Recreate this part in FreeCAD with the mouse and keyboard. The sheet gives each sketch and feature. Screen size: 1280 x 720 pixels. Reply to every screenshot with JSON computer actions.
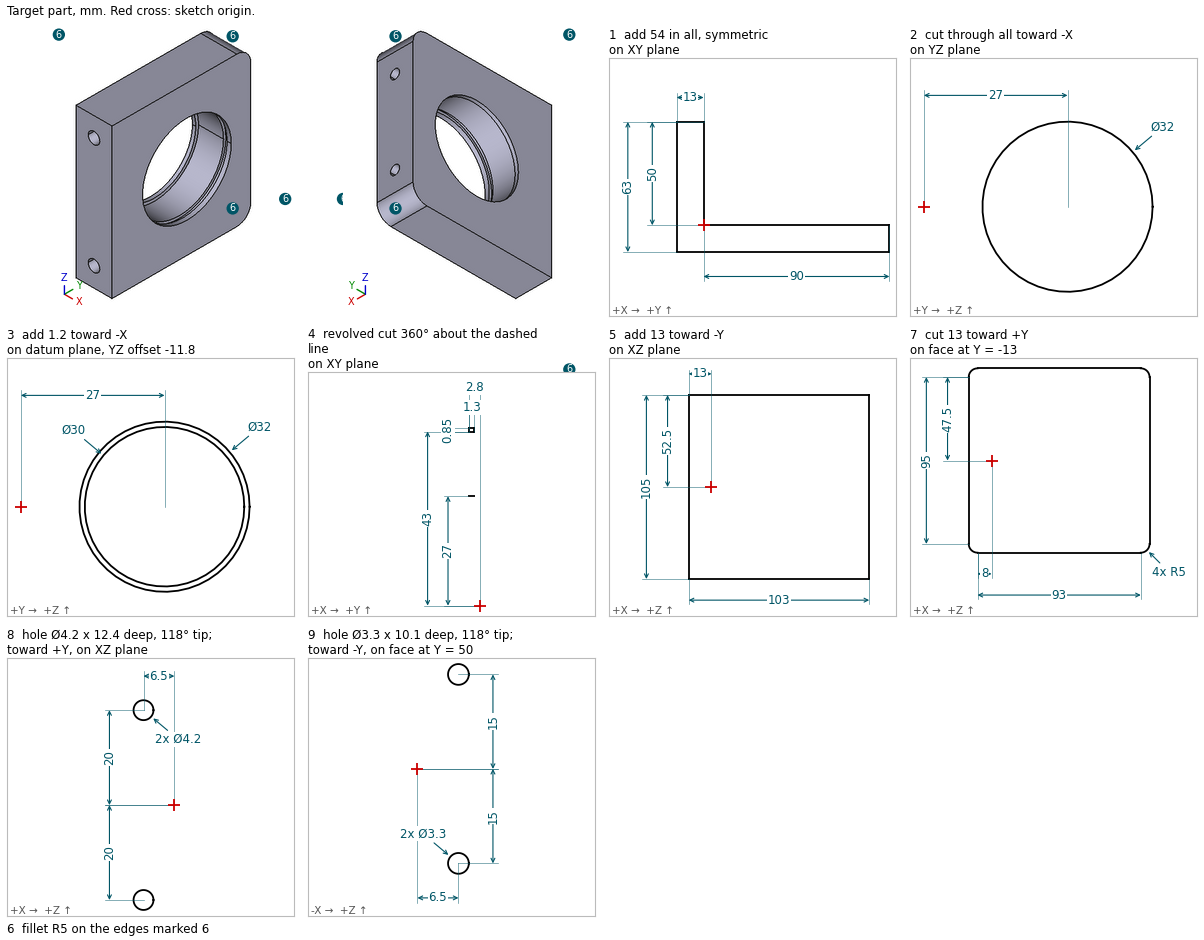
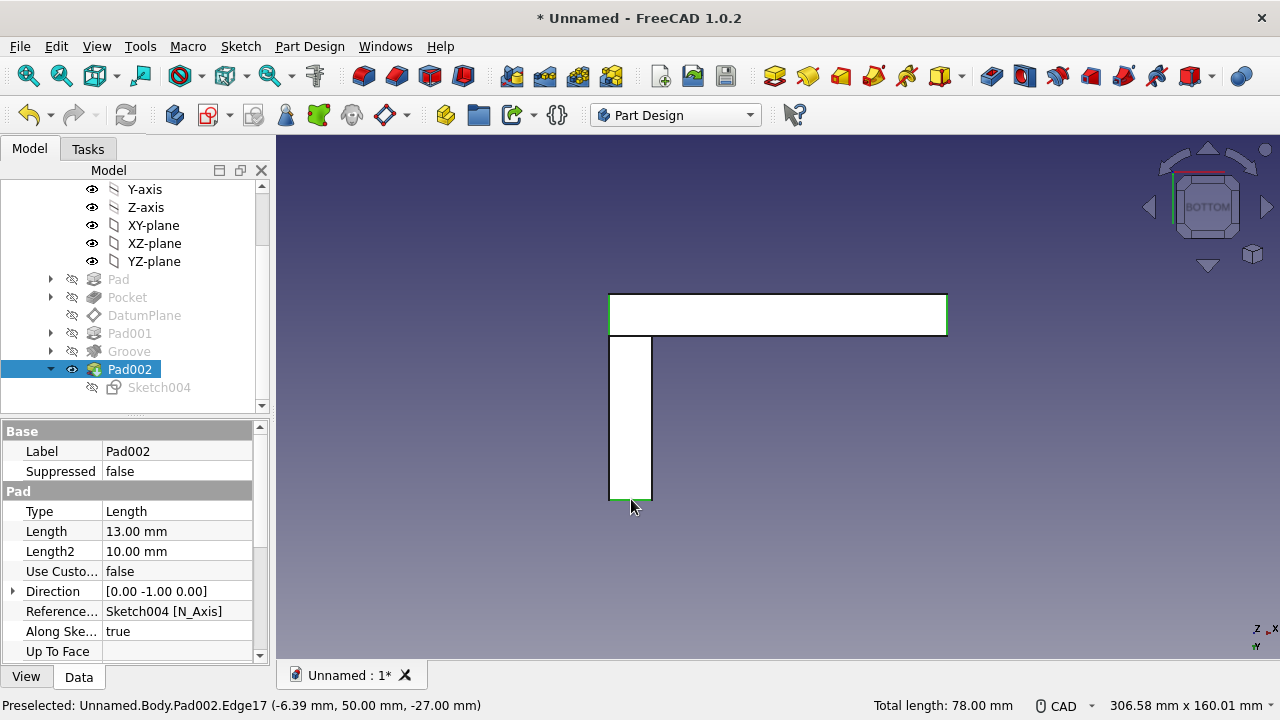
{"action": "left_click", "coordinate": [364, 76]}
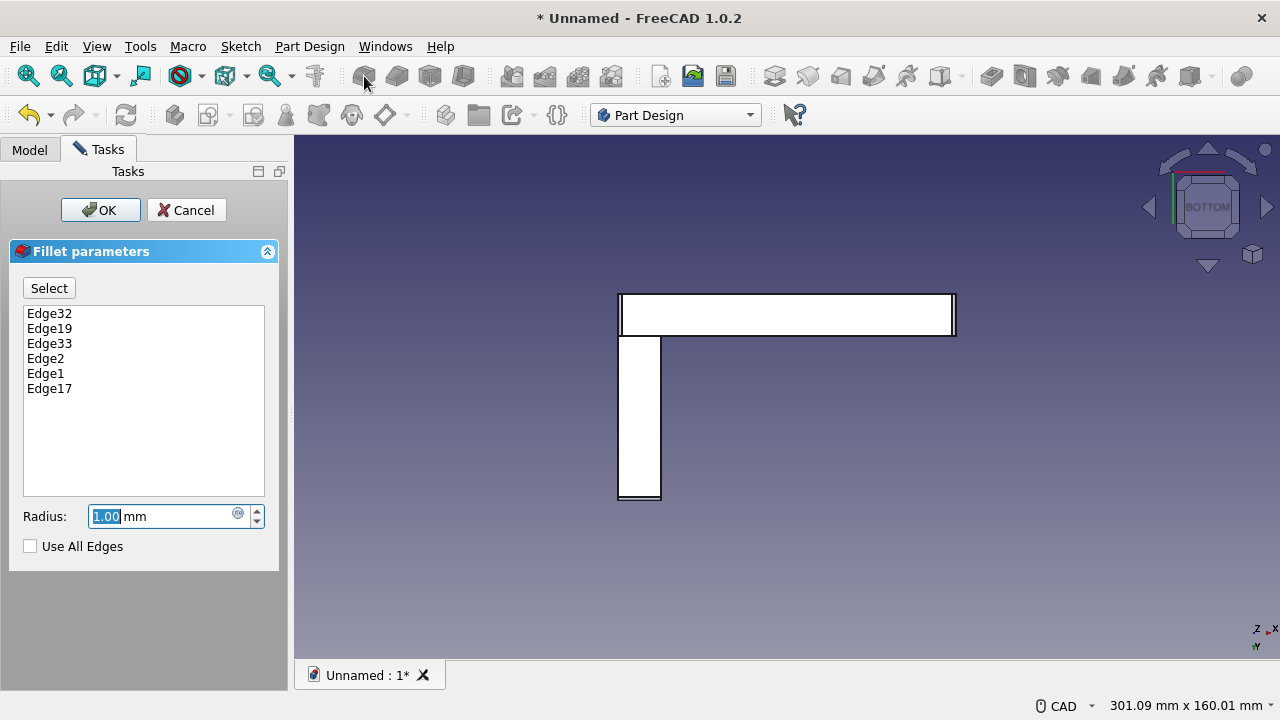
{"action": "type", "text": "5"}
{"action": "key", "text": "Tab"}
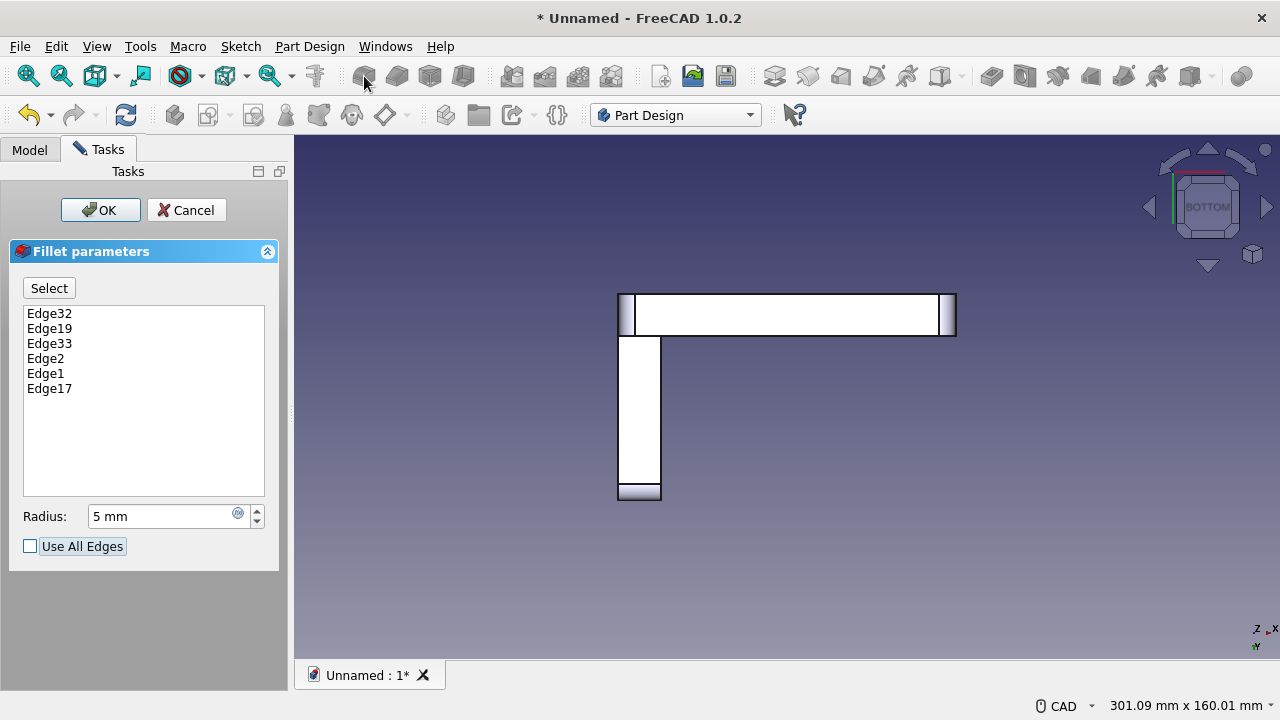
{"action": "left_click", "coordinate": [101, 210]}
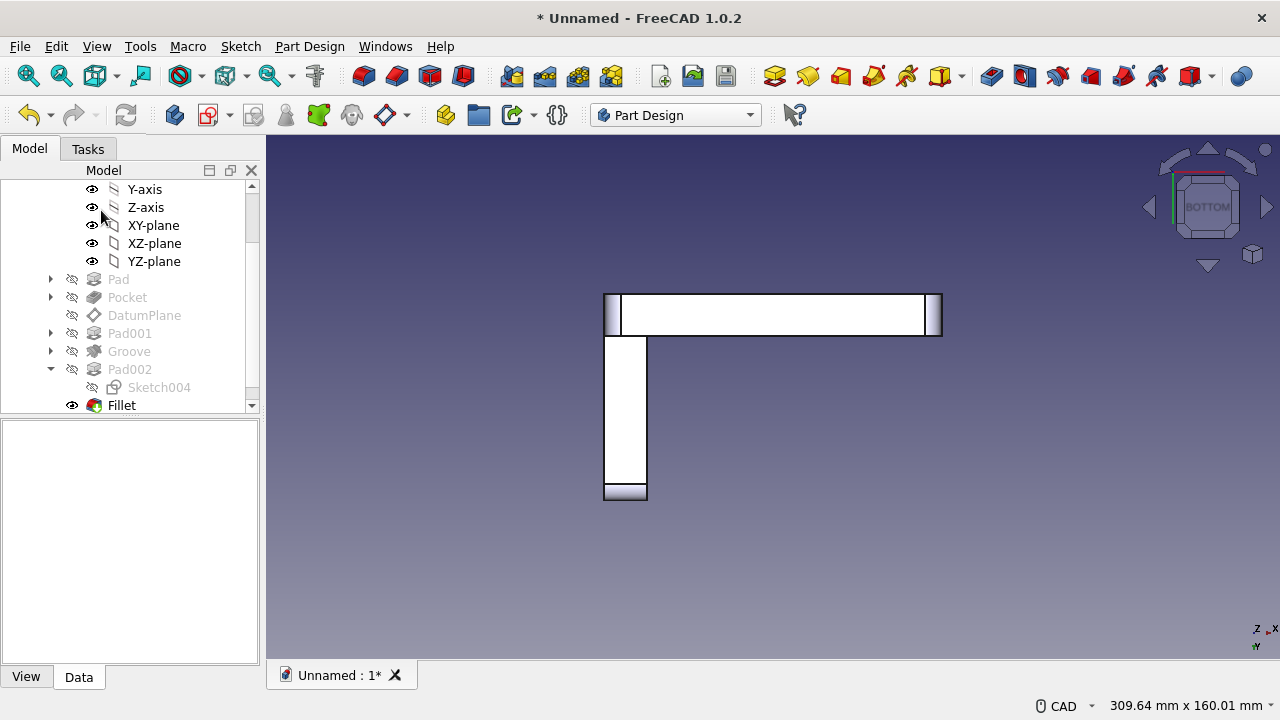
{"action": "left_click", "coordinate": [29, 76]}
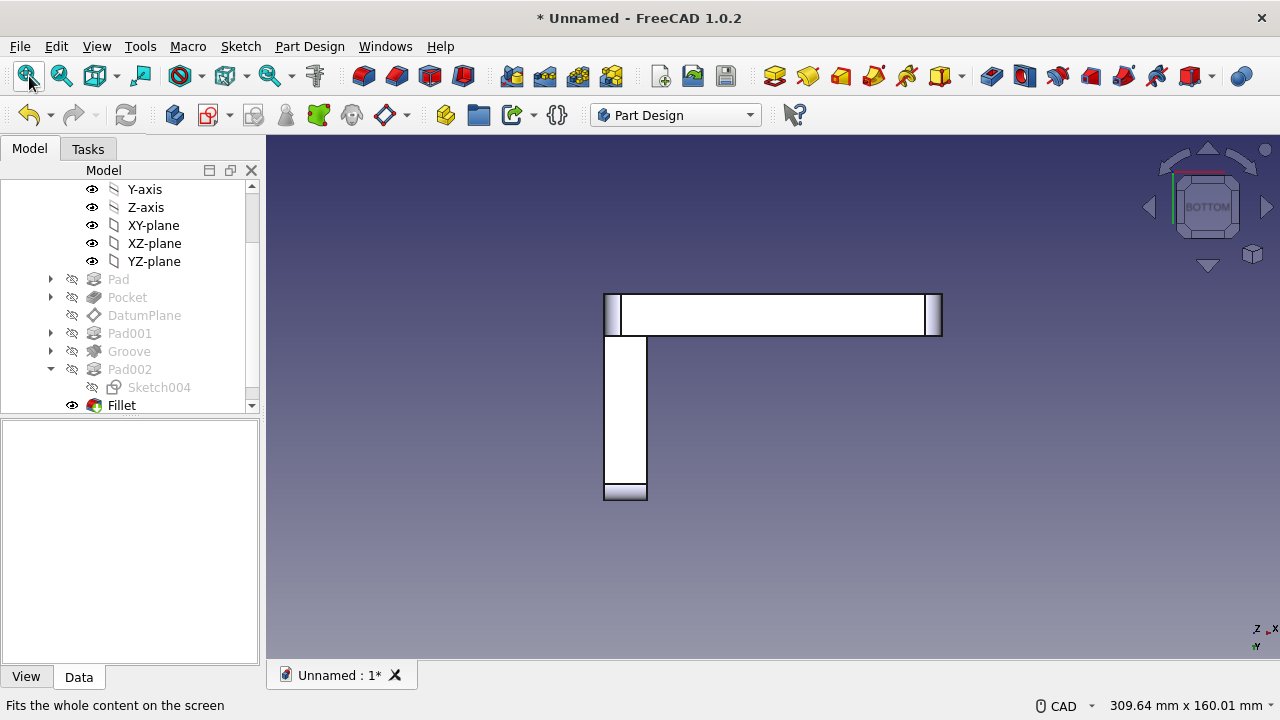
{"action": "key", "text": "0"}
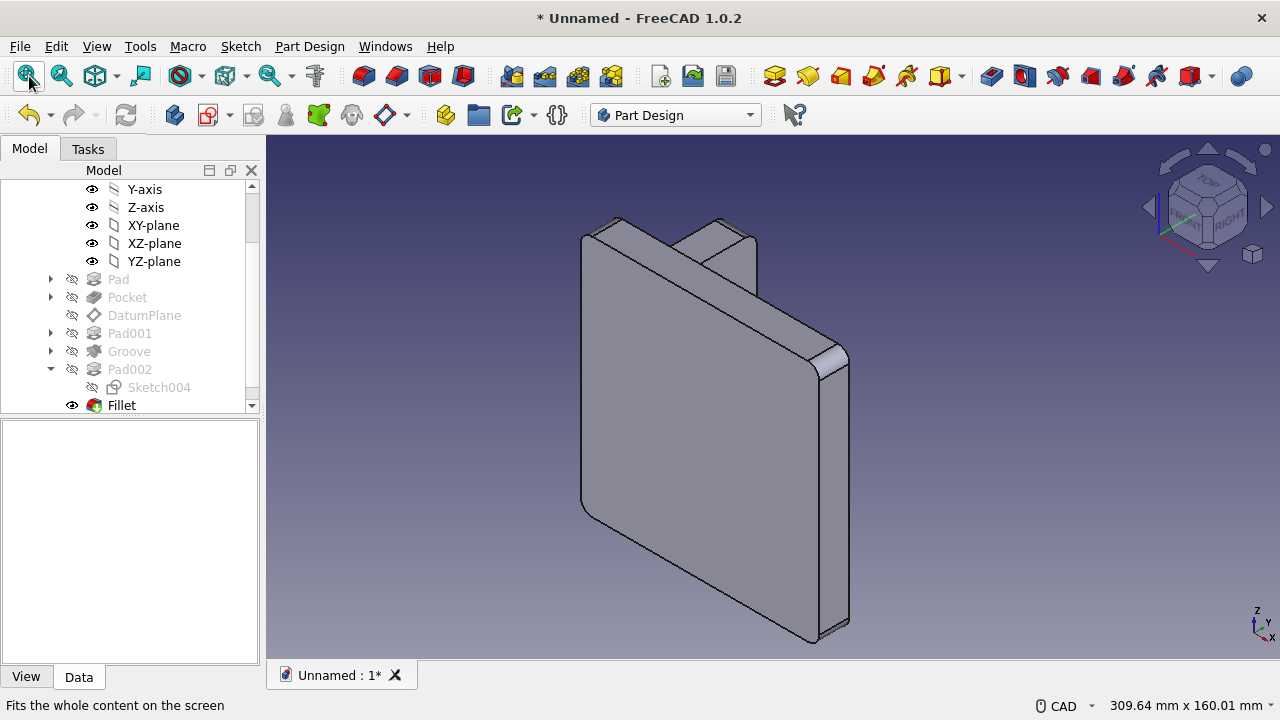
{"action": "left_click", "coordinate": [700, 438]}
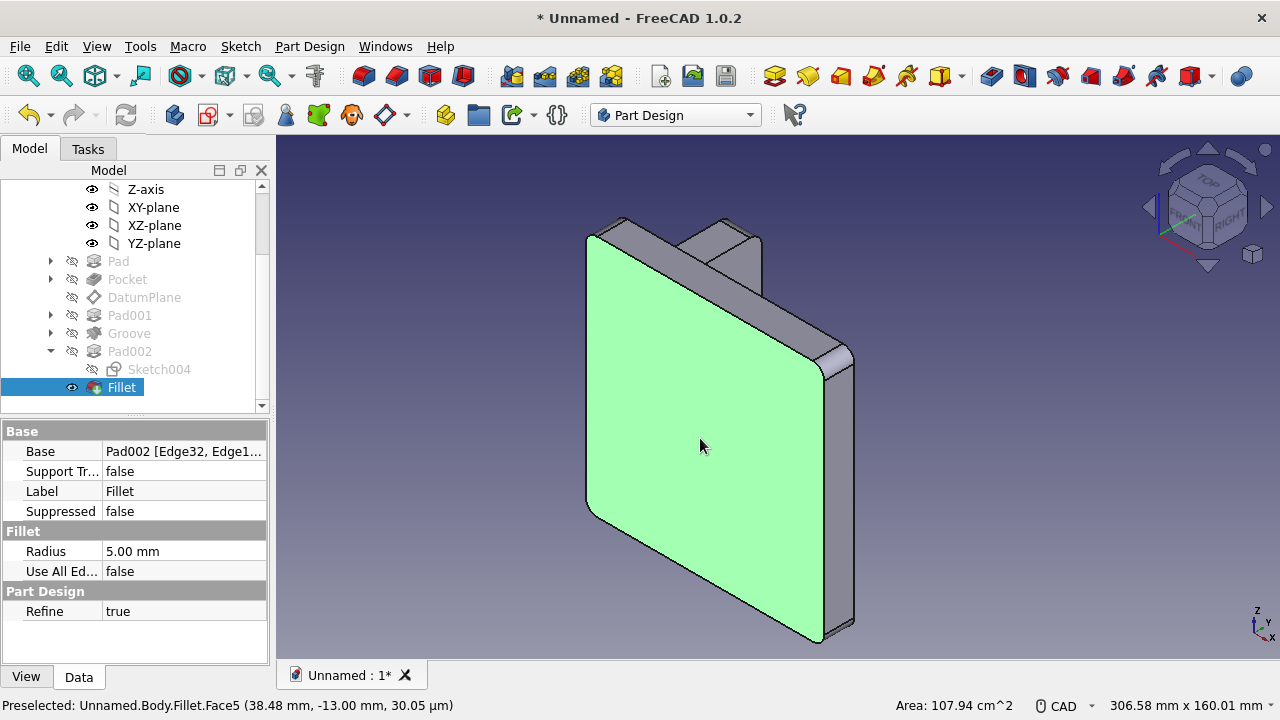
{"action": "left_click", "coordinate": [208, 116]}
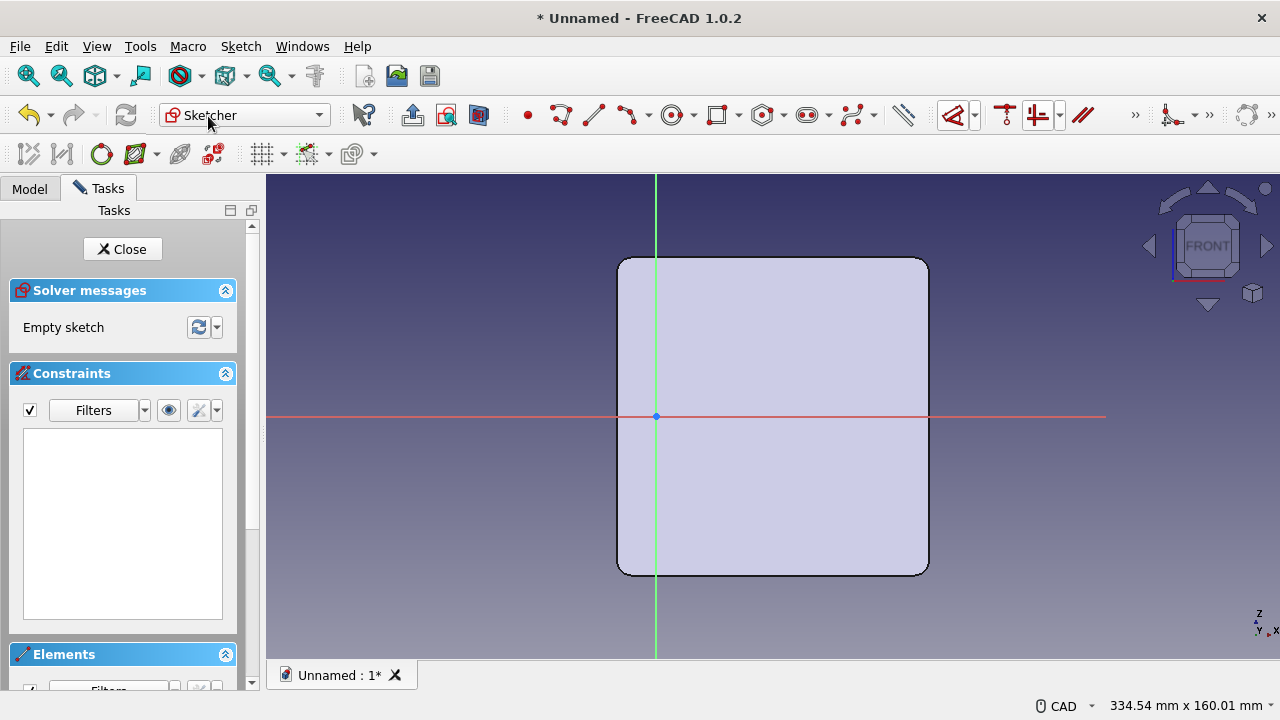
{"action": "left_click", "coordinate": [594, 116]}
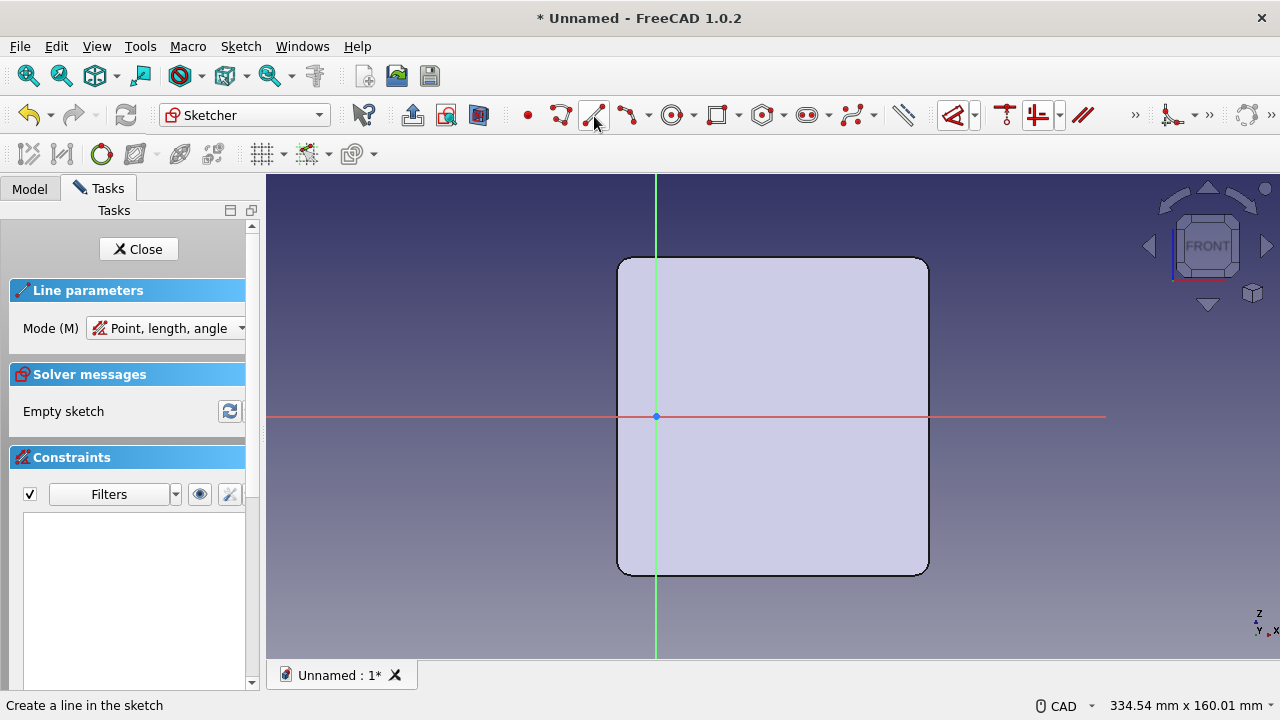
{"action": "left_click", "coordinate": [617, 273]}
{"action": "left_click", "coordinate": [617, 560]}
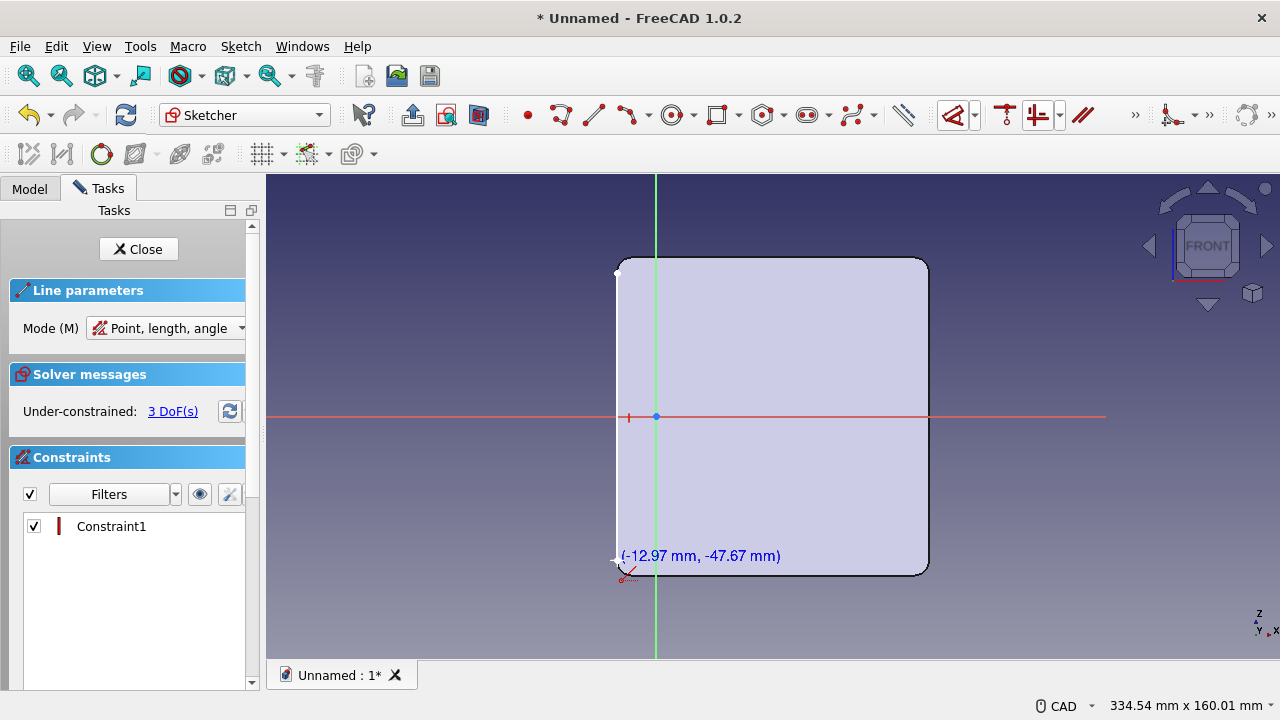
{"action": "left_click", "coordinate": [632, 576]}
{"action": "left_click", "coordinate": [914, 576]}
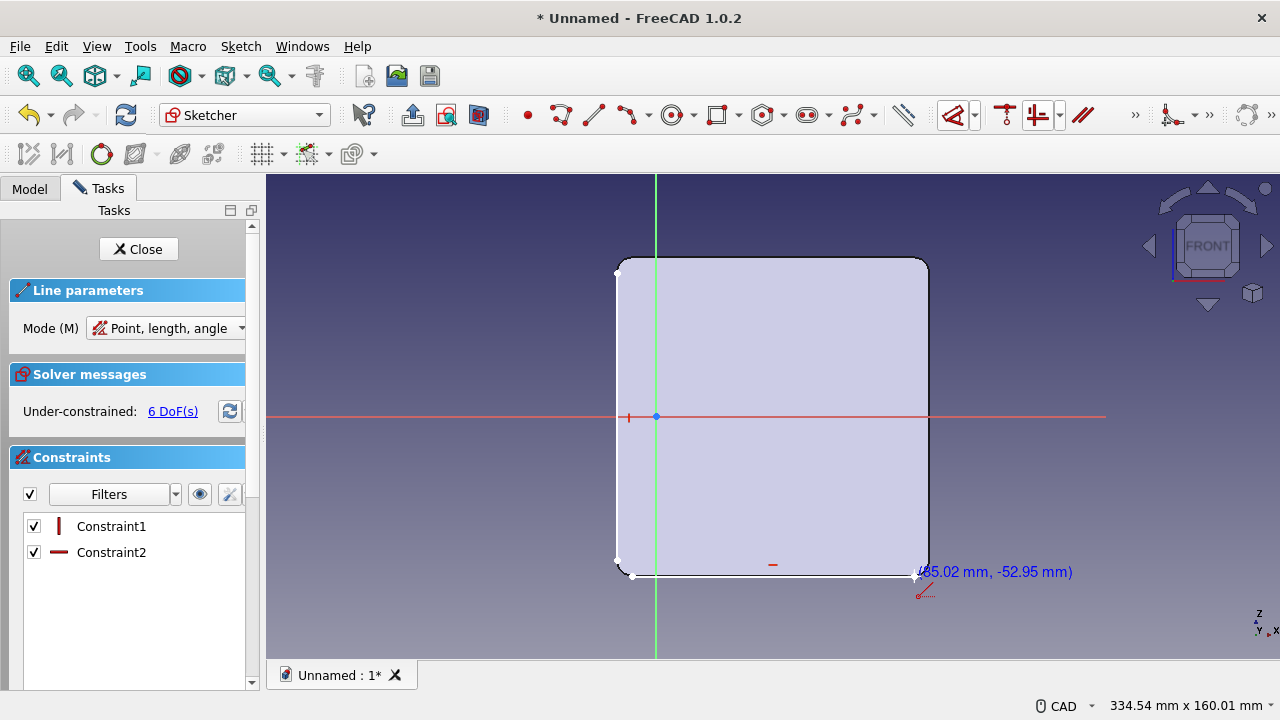
{"action": "left_click", "coordinate": [929, 560]}
{"action": "left_click", "coordinate": [929, 273]}